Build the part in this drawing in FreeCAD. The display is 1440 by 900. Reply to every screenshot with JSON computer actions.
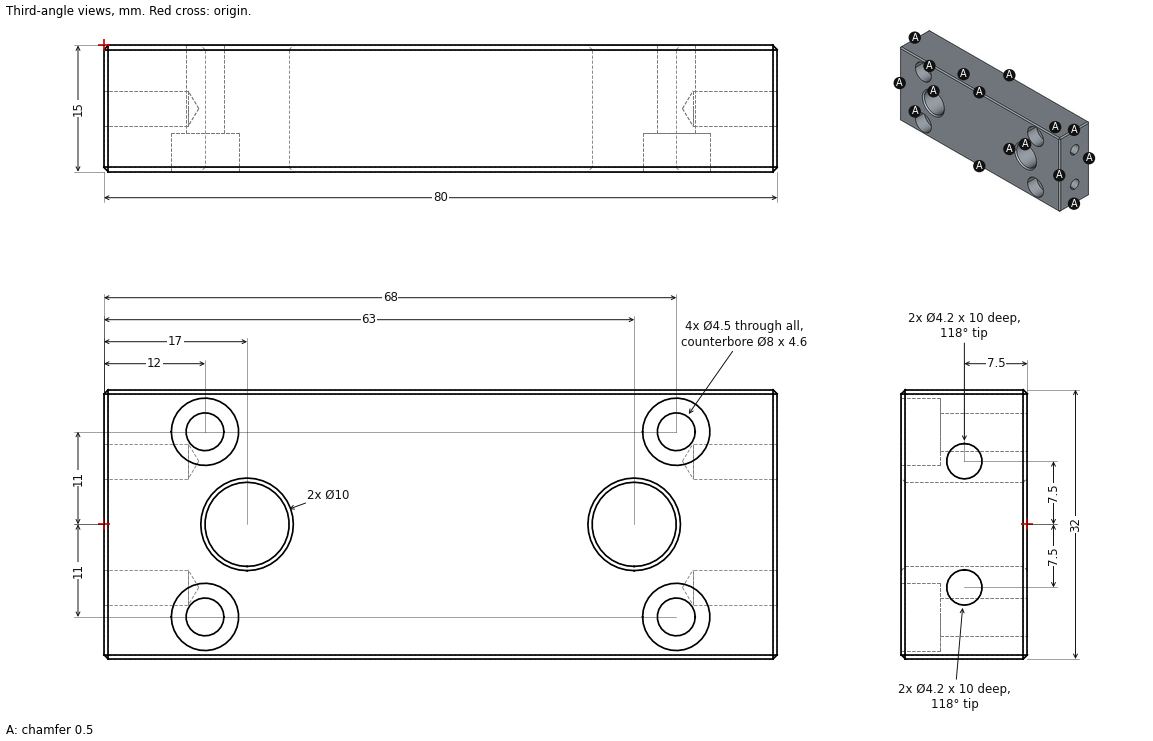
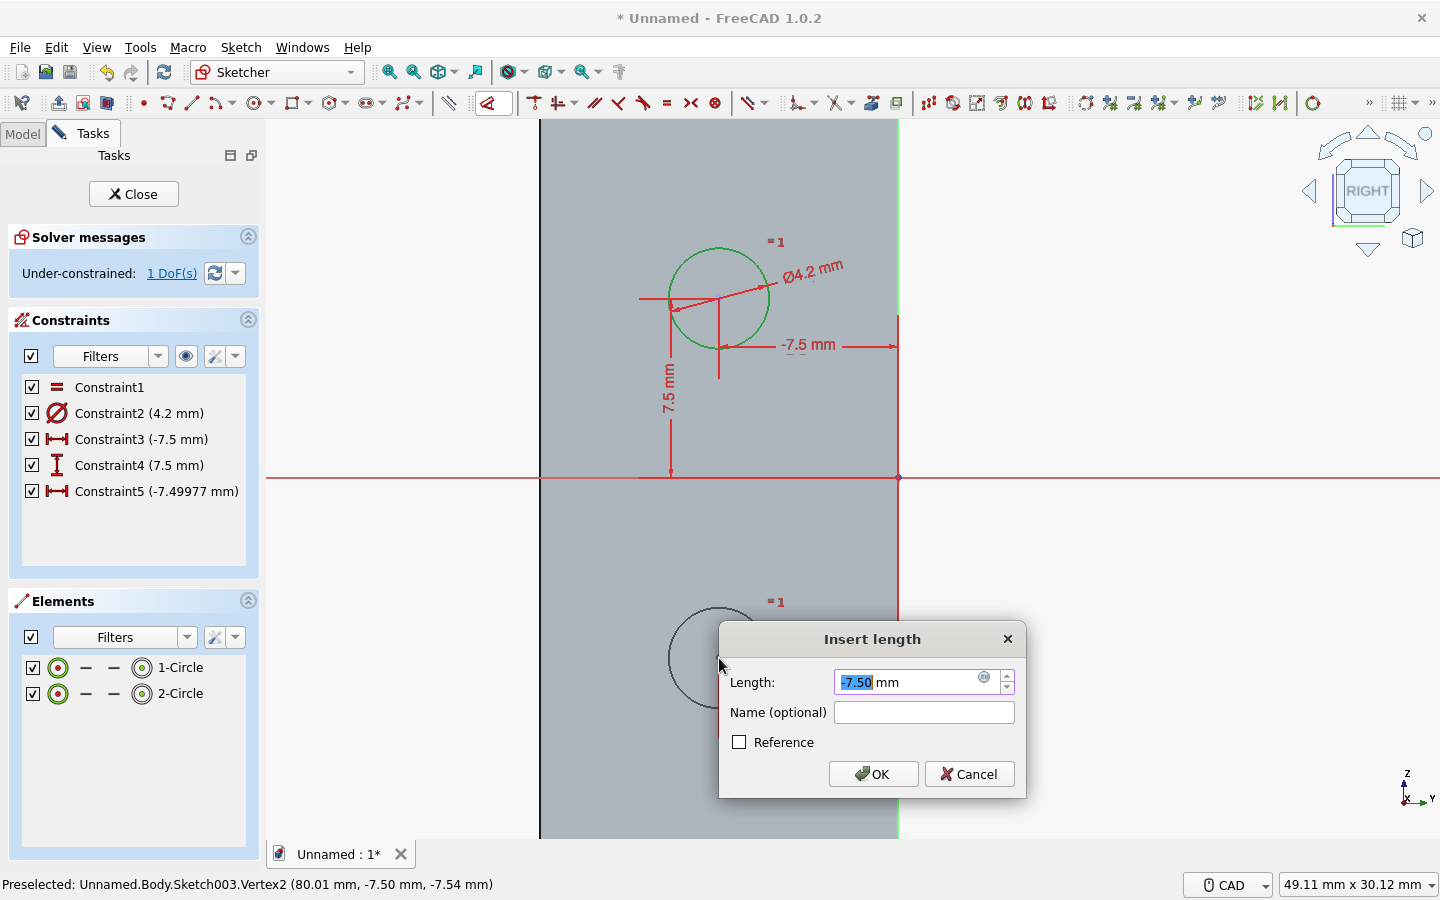
{"action": "type", "text": "-7.5"}
{"action": "key", "text": "Return"}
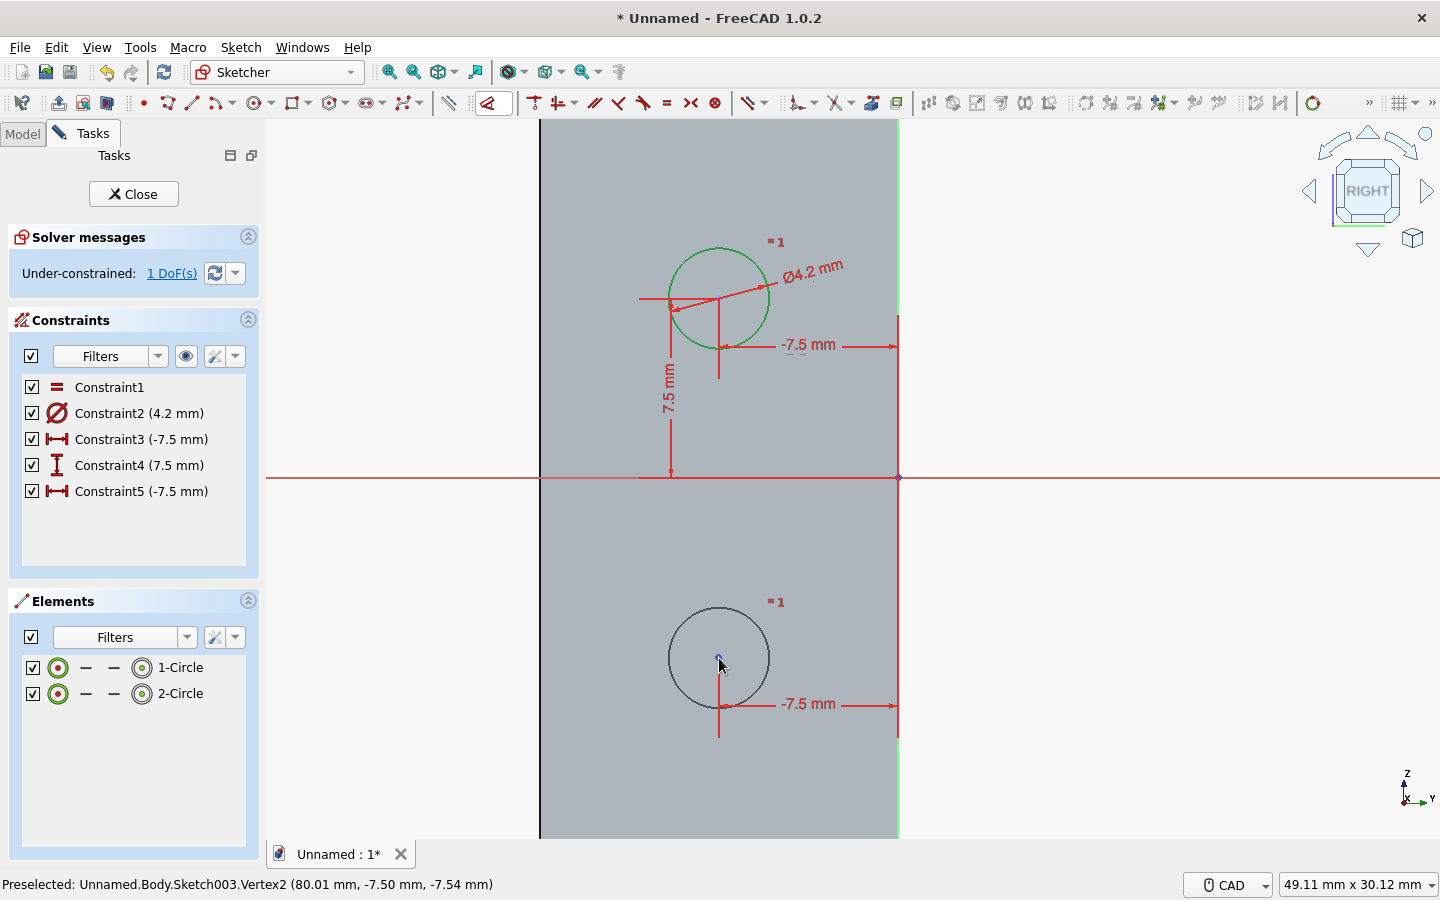
{"action": "left_click", "coordinate": [719, 658]}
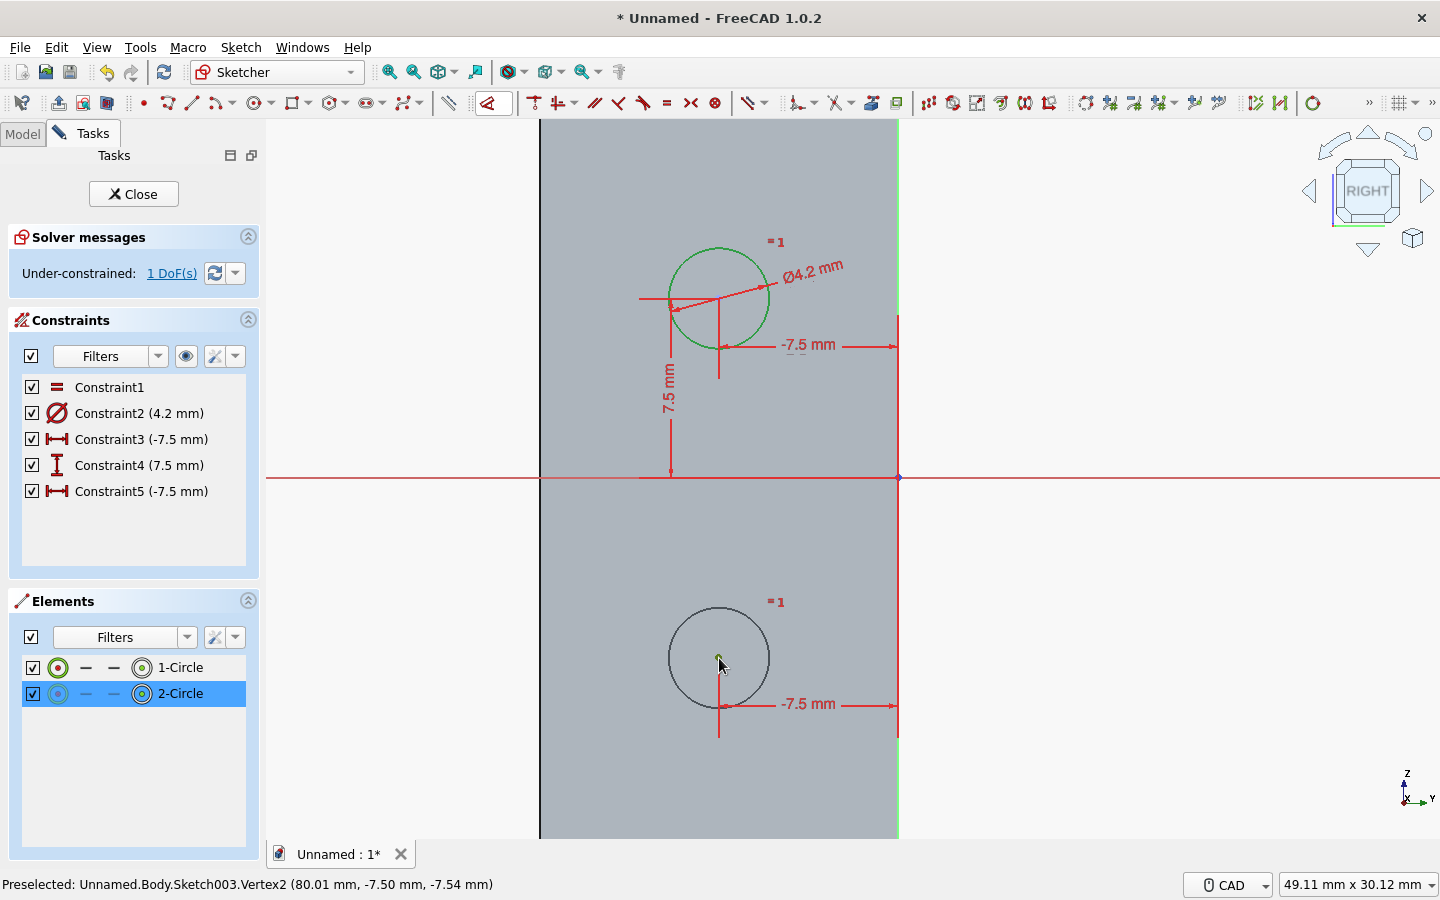
{"action": "key", "text": "i"}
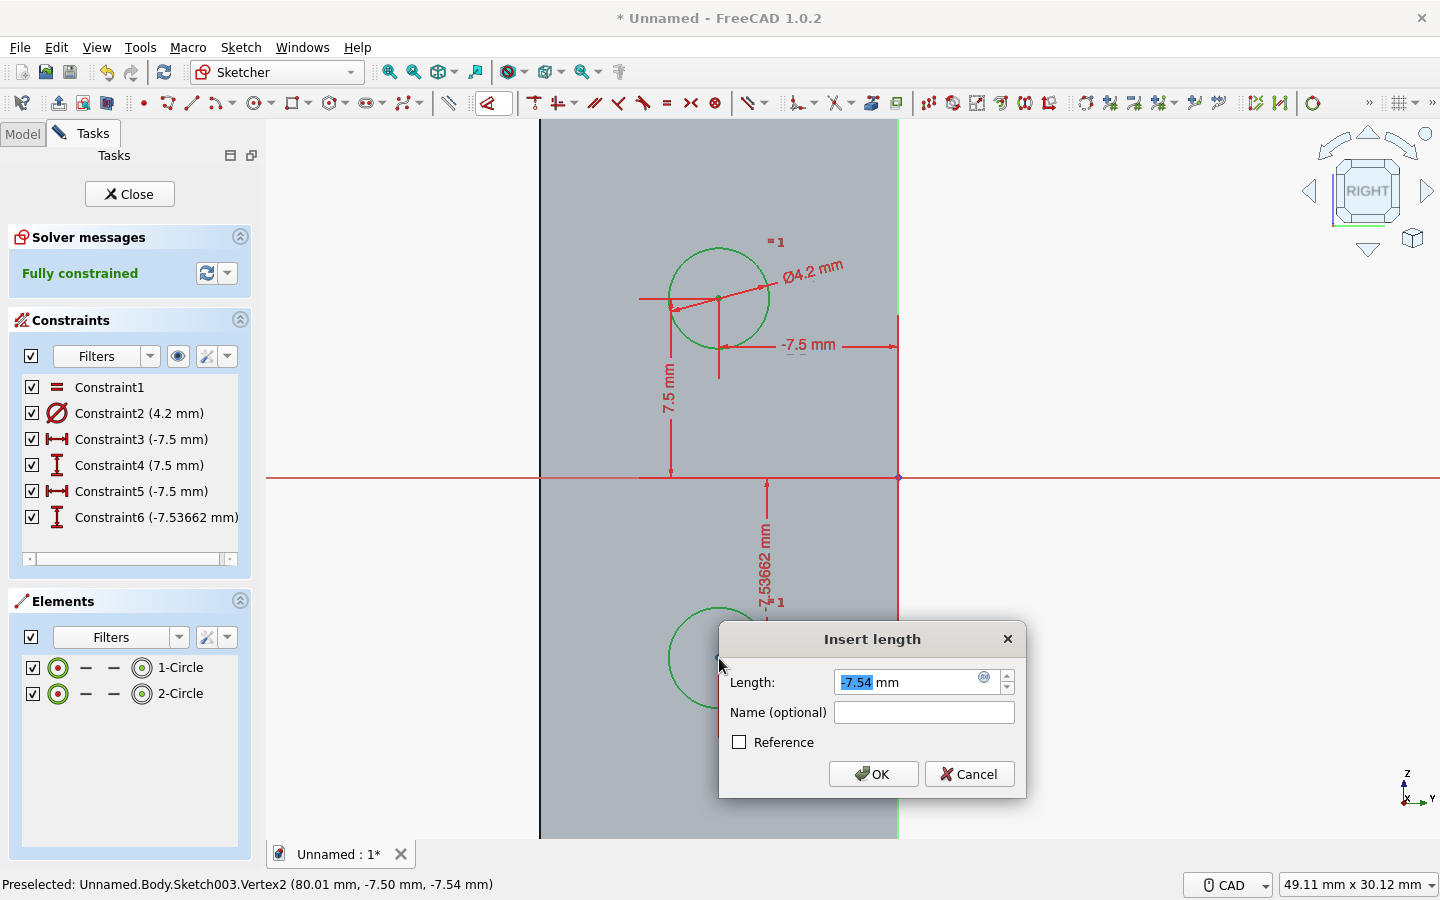
{"action": "type", "text": "-7.5"}
{"action": "key", "text": "Return"}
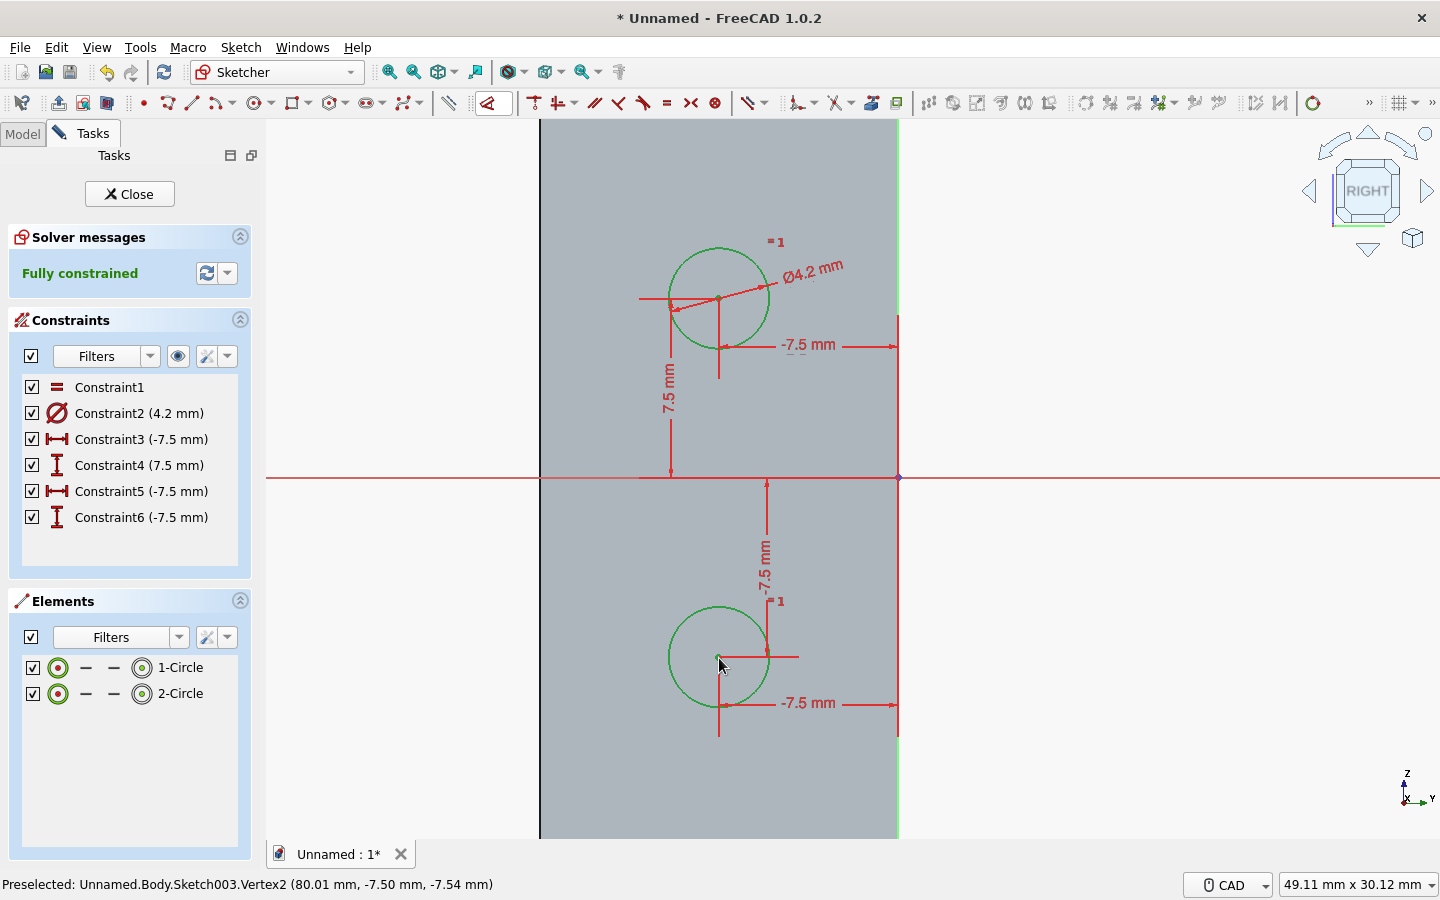
{"action": "left_click", "coordinate": [130, 194]}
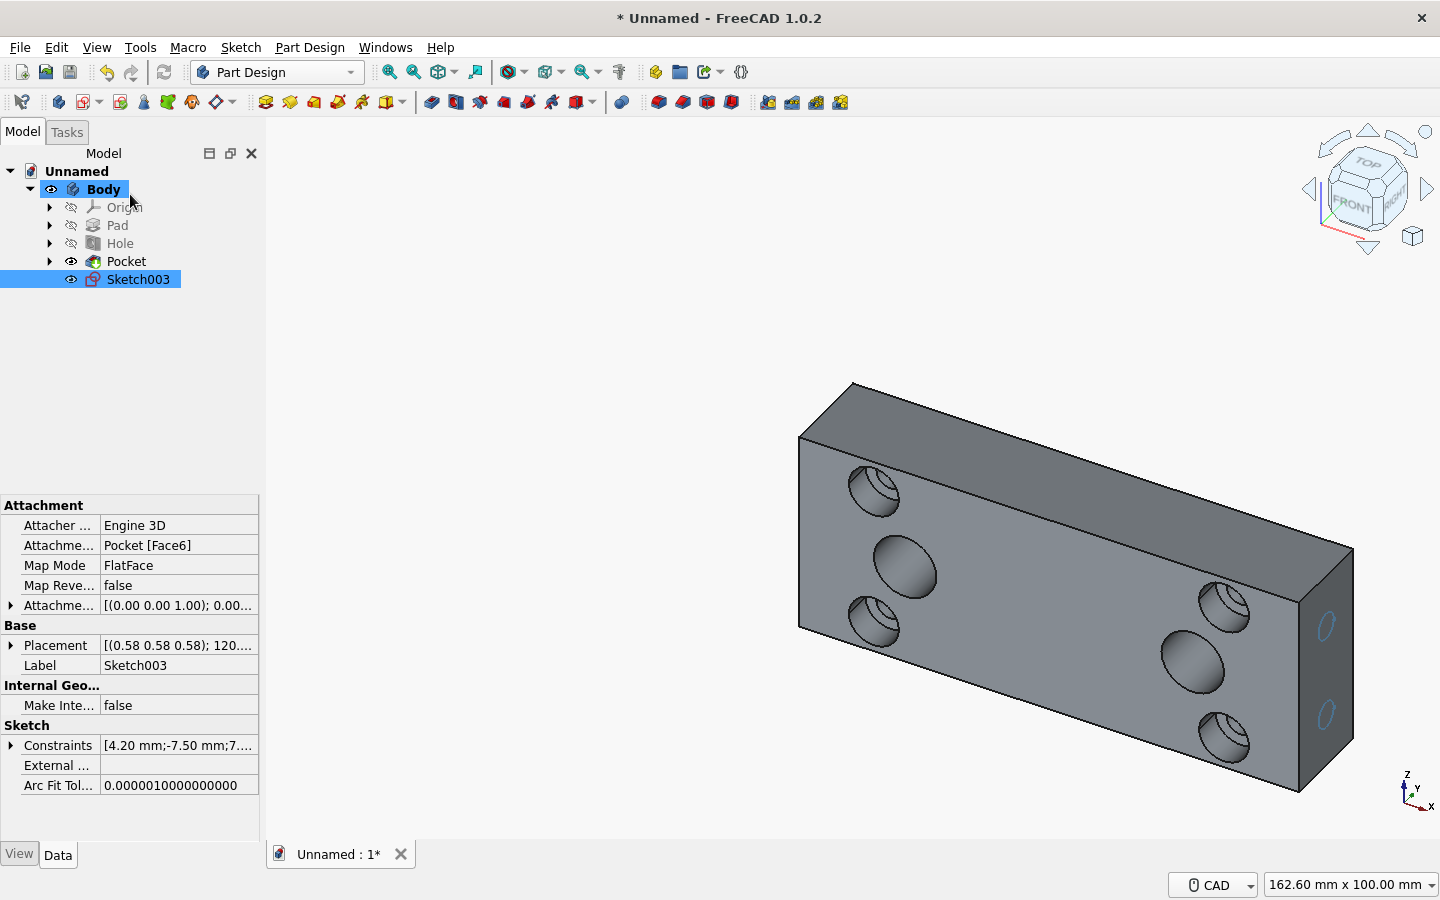
{"action": "left_click", "coordinate": [456, 102]}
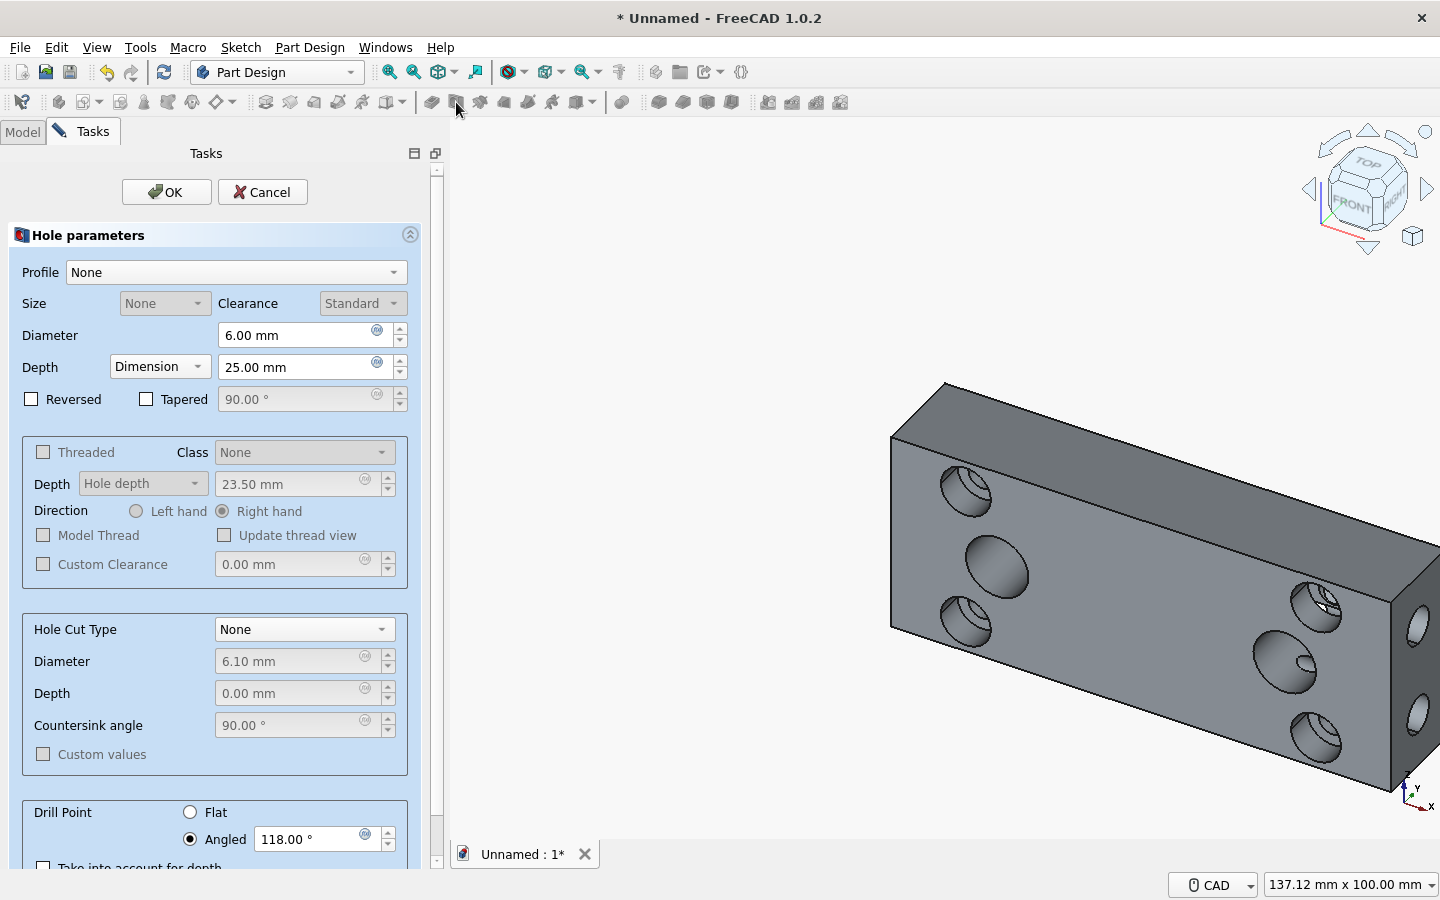
{"action": "triple_click", "coordinate": [305, 335]}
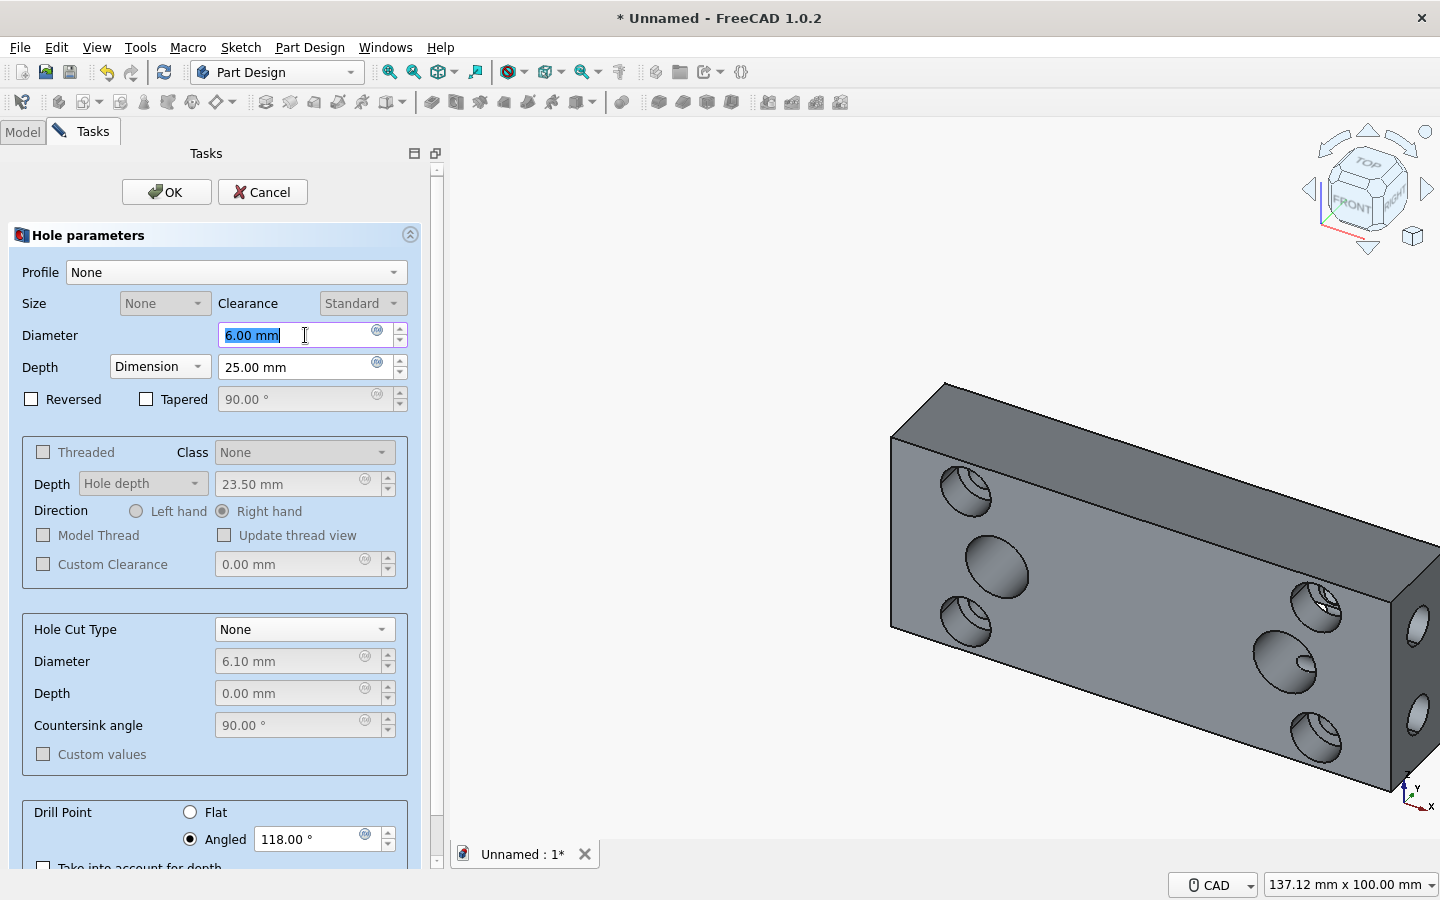
{"action": "type", "text": "4.2"}
{"action": "key", "text": "Tab"}